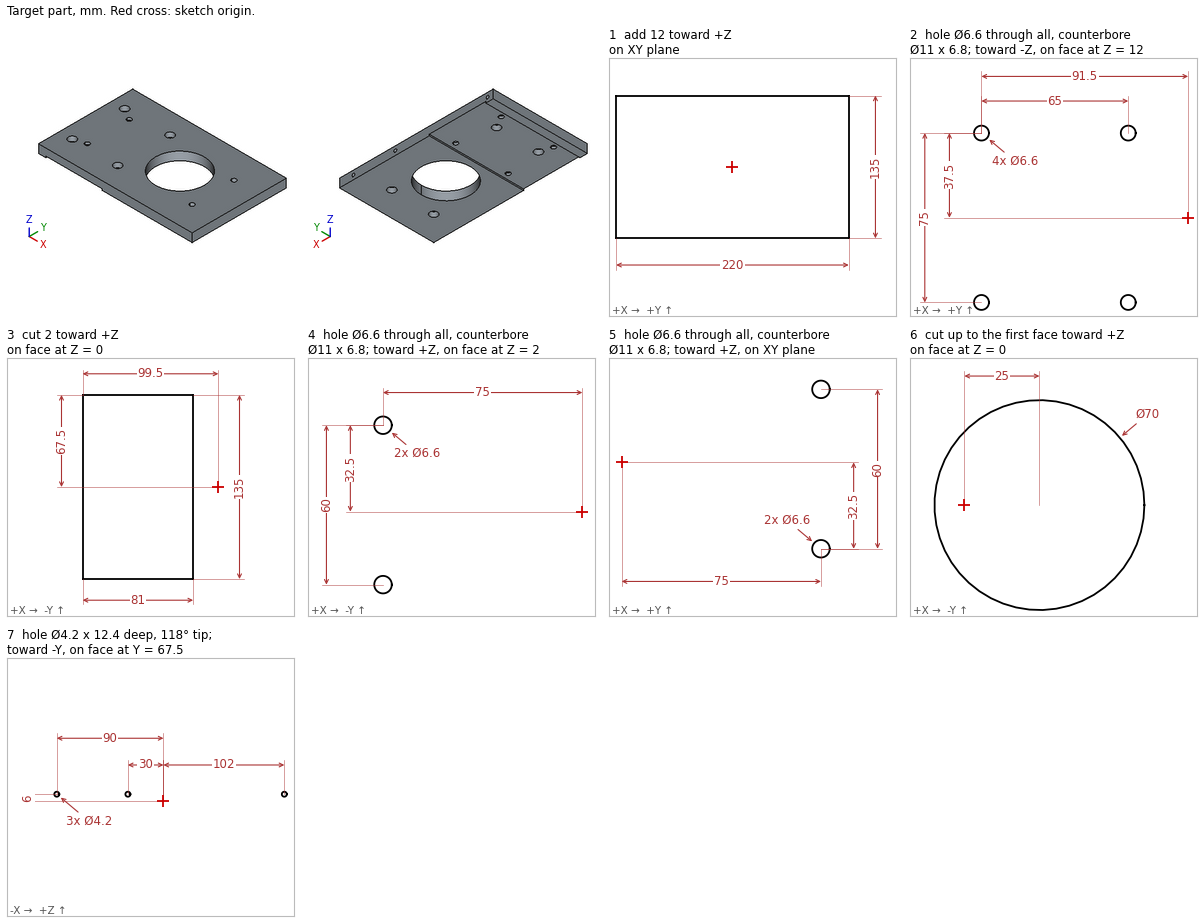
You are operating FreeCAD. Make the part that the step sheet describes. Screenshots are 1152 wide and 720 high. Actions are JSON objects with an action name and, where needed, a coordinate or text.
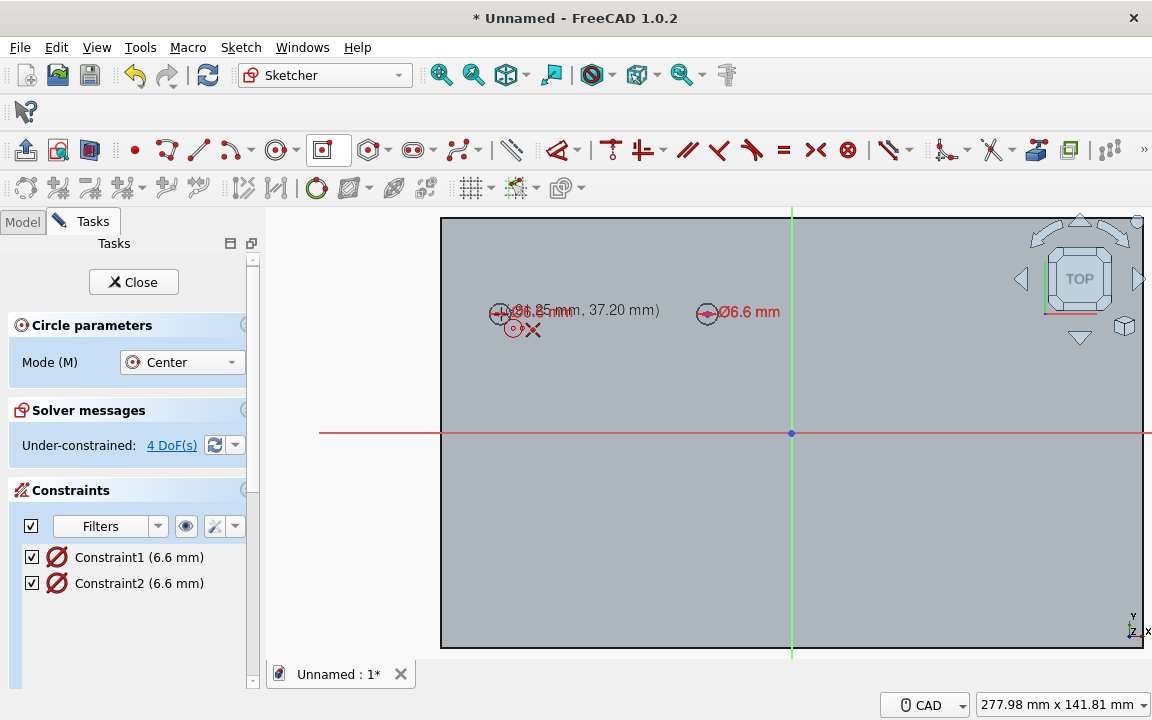
{"action": "scroll", "coordinate": [500, 553], "scroll_direction": "up", "scroll_amount": 4}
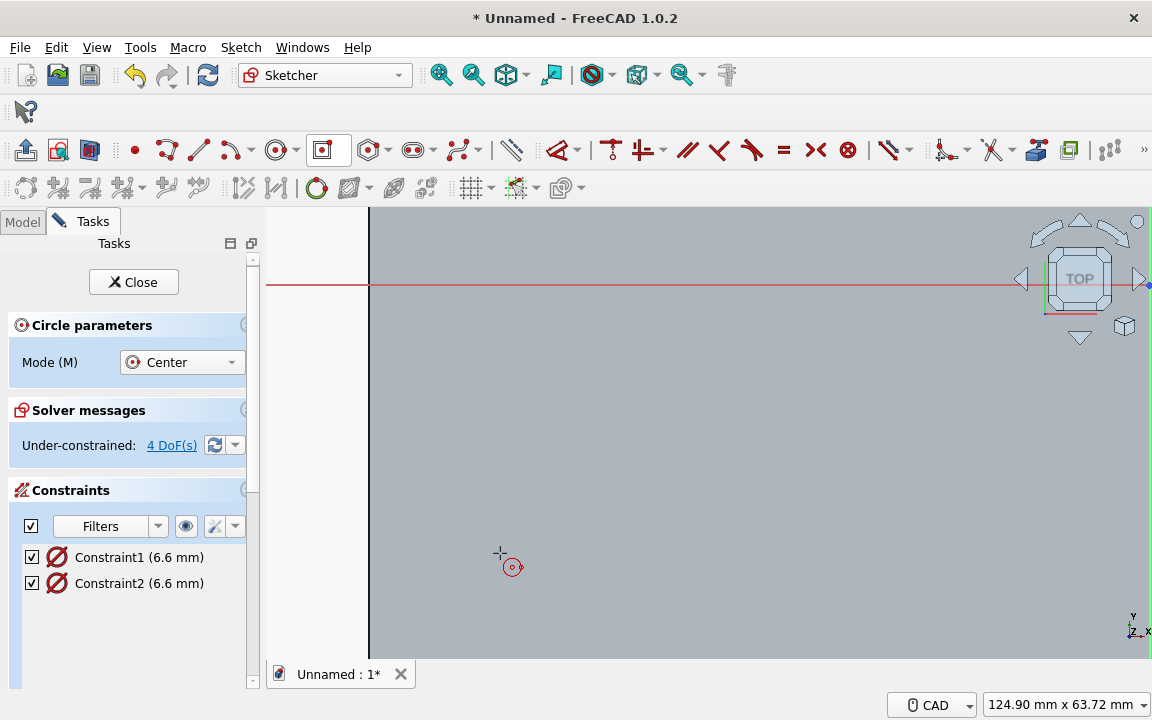
{"action": "left_click", "coordinate": [500, 551]}
{"action": "mouse_move", "coordinate": [517, 535]}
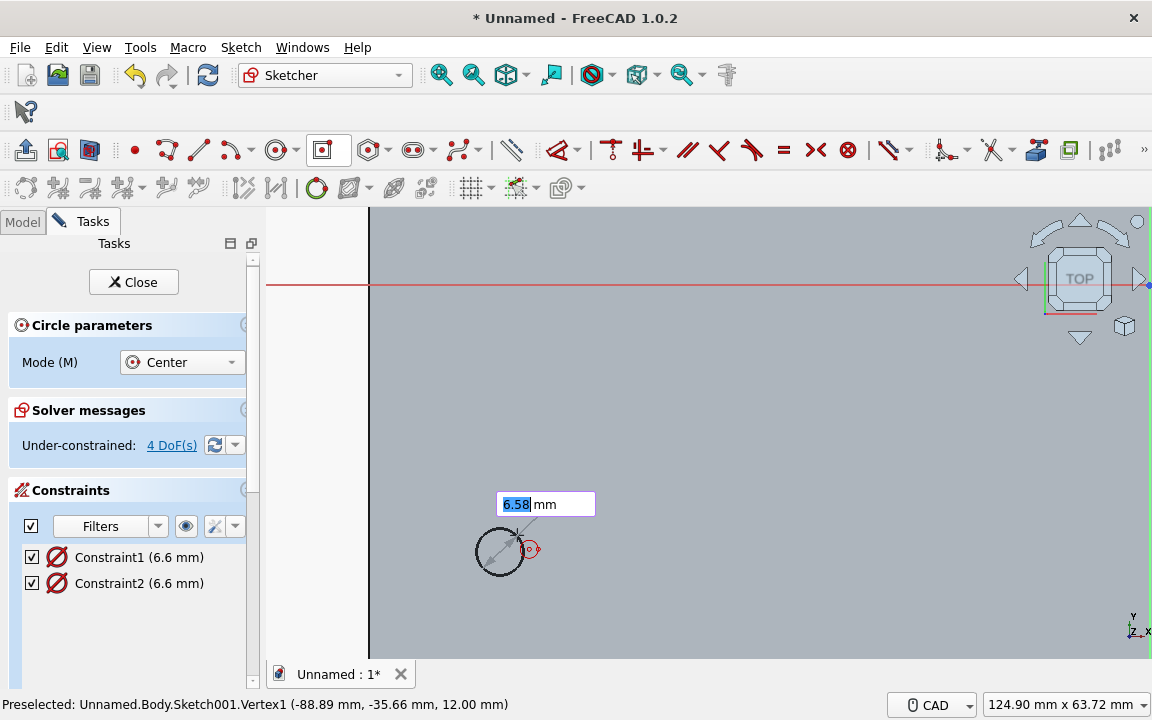
{"action": "type", "text": "6.6"}
{"action": "key", "text": "Return"}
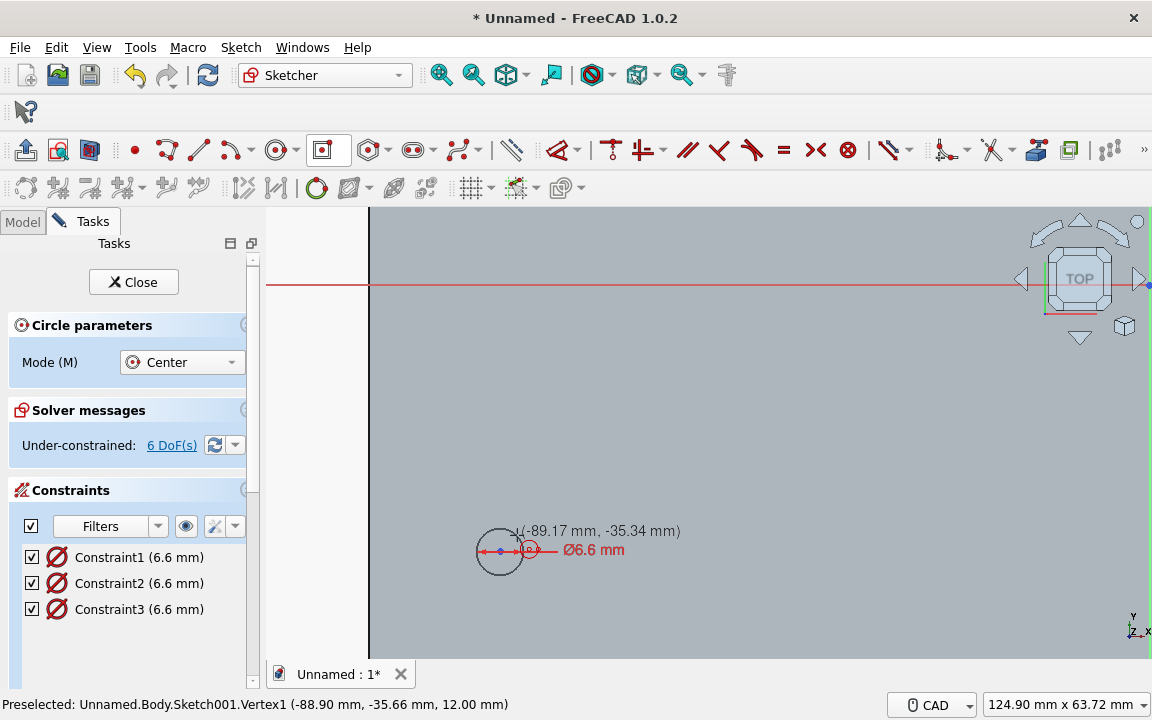
{"action": "left_click", "coordinate": [962, 551]}
{"action": "mouse_move", "coordinate": [978, 535]}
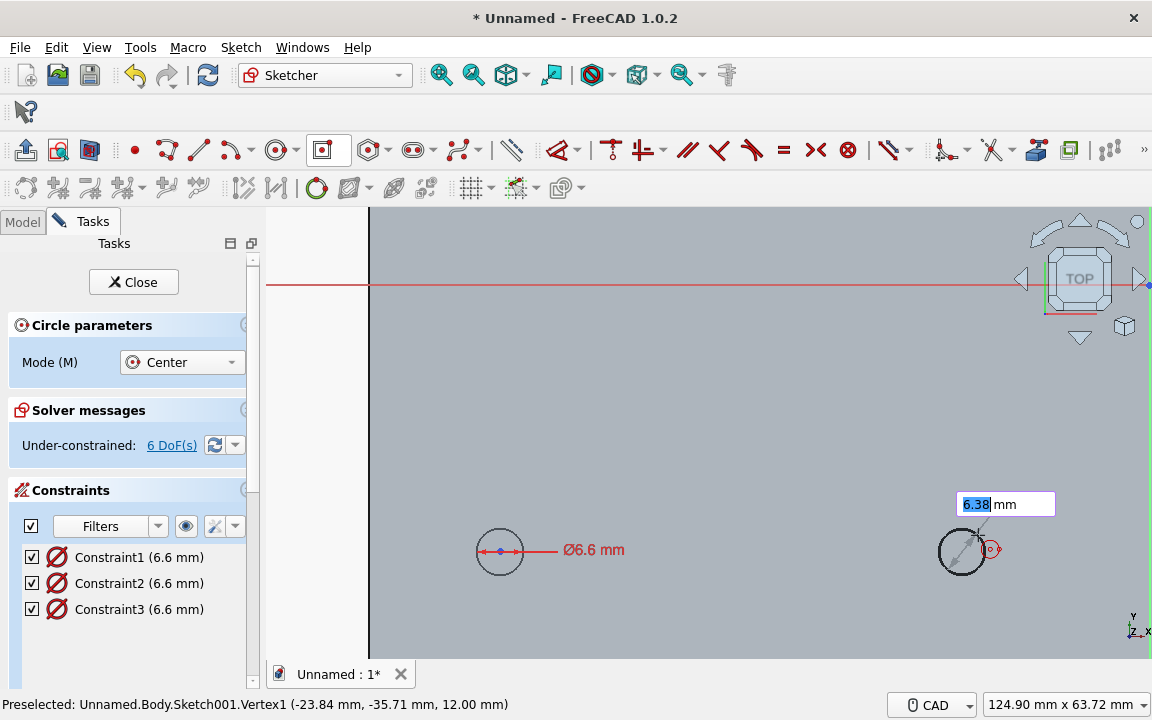
{"action": "type", "text": "6.6"}
{"action": "key", "text": "Return"}
{"action": "key", "text": "Escape"}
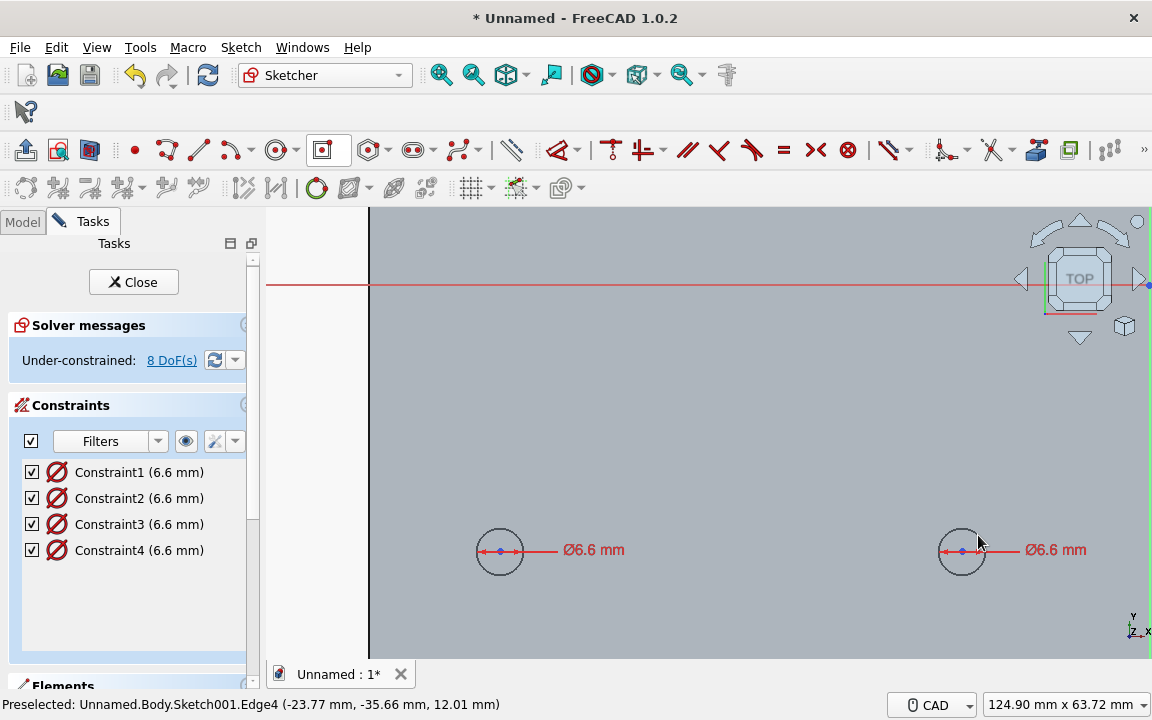
{"action": "scroll", "coordinate": [500, 554], "scroll_direction": "down", "scroll_amount": 4}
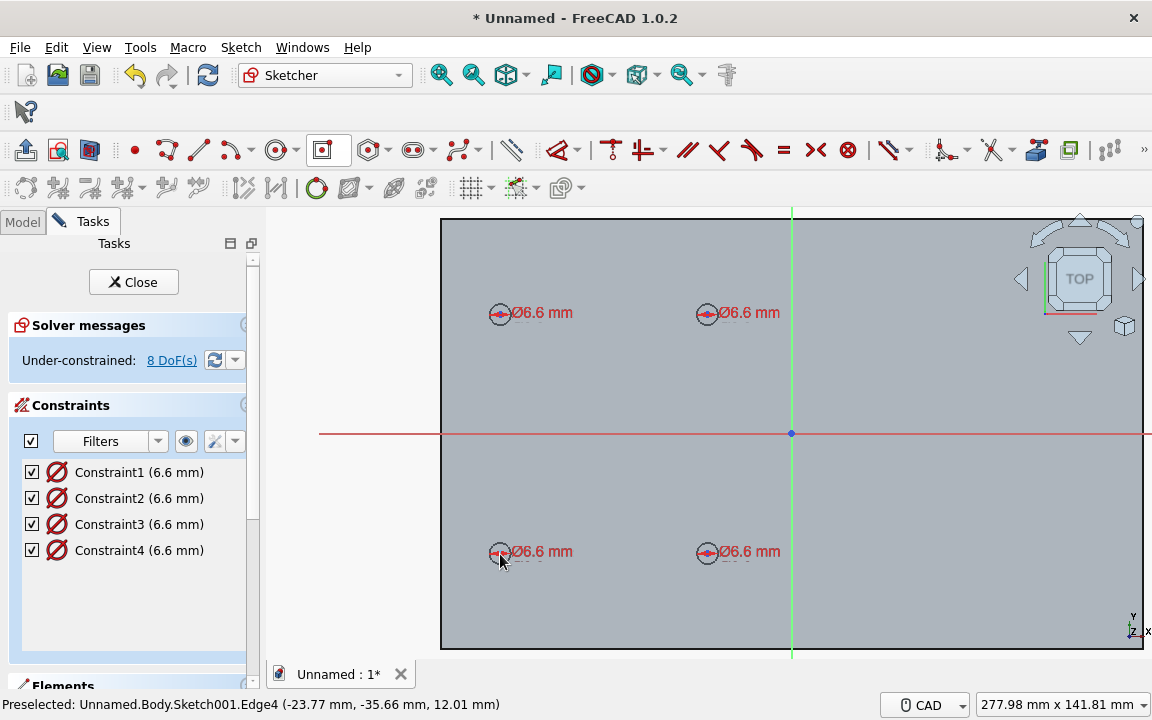
{"action": "left_click", "coordinate": [500, 315]}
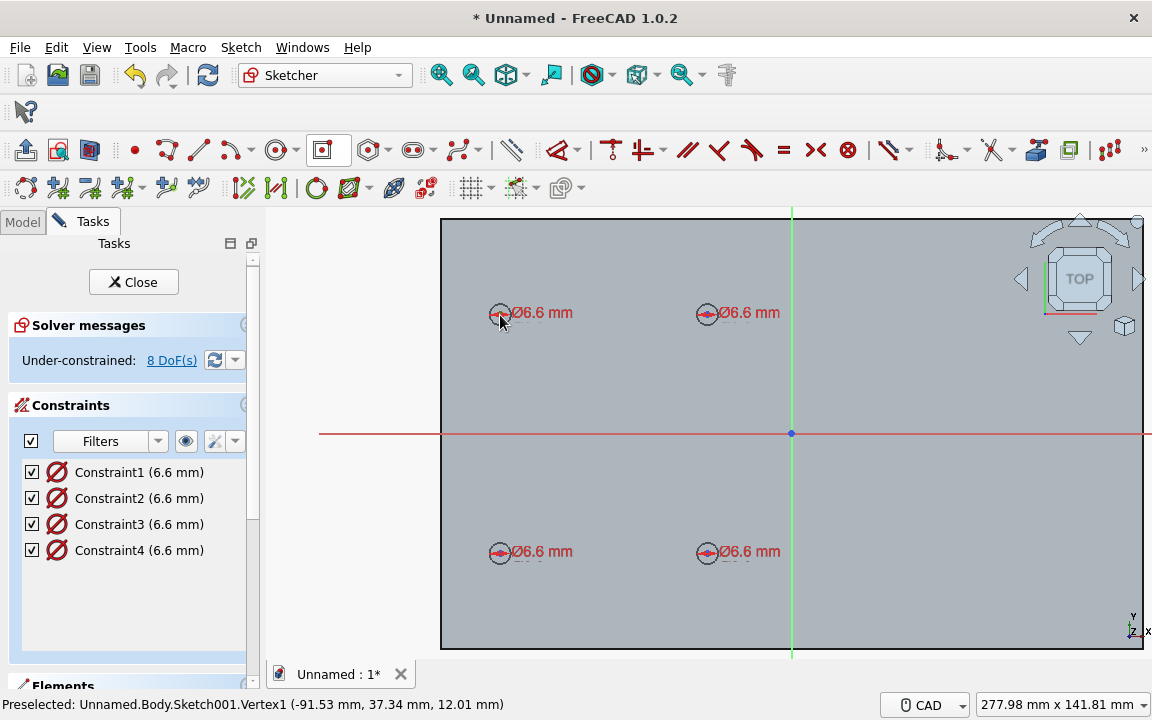
{"action": "left_click", "coordinate": [707, 315]}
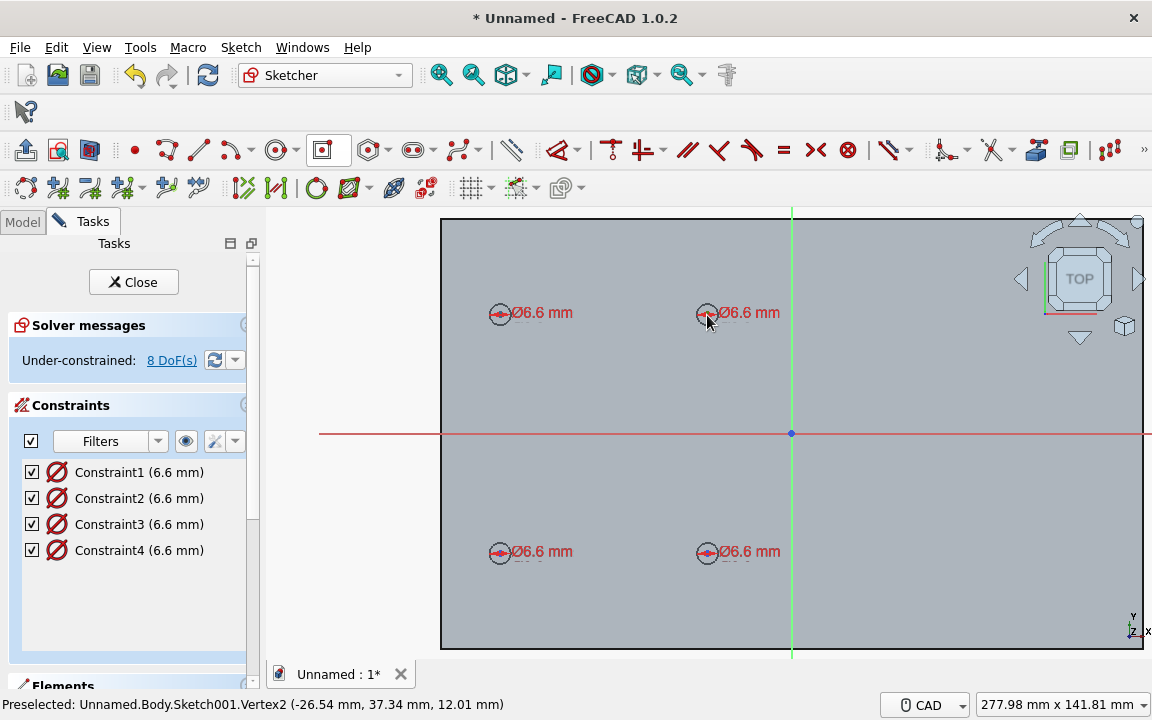
{"action": "key", "text": "h"}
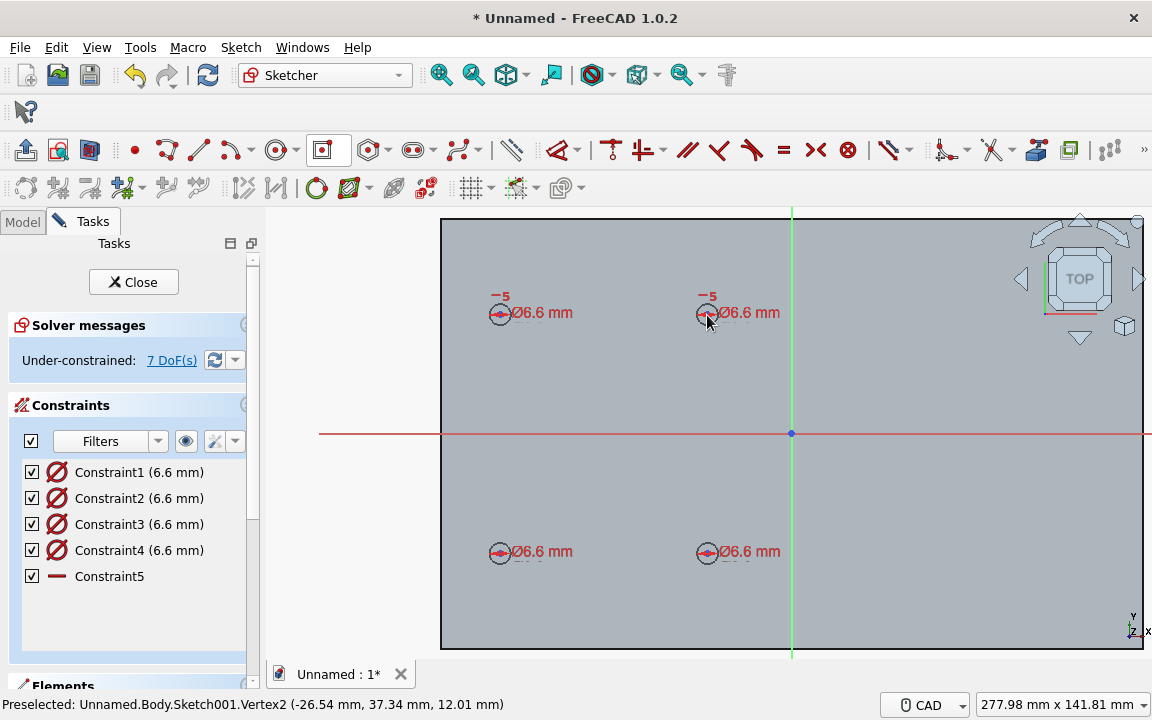
{"action": "left_click", "coordinate": [500, 315]}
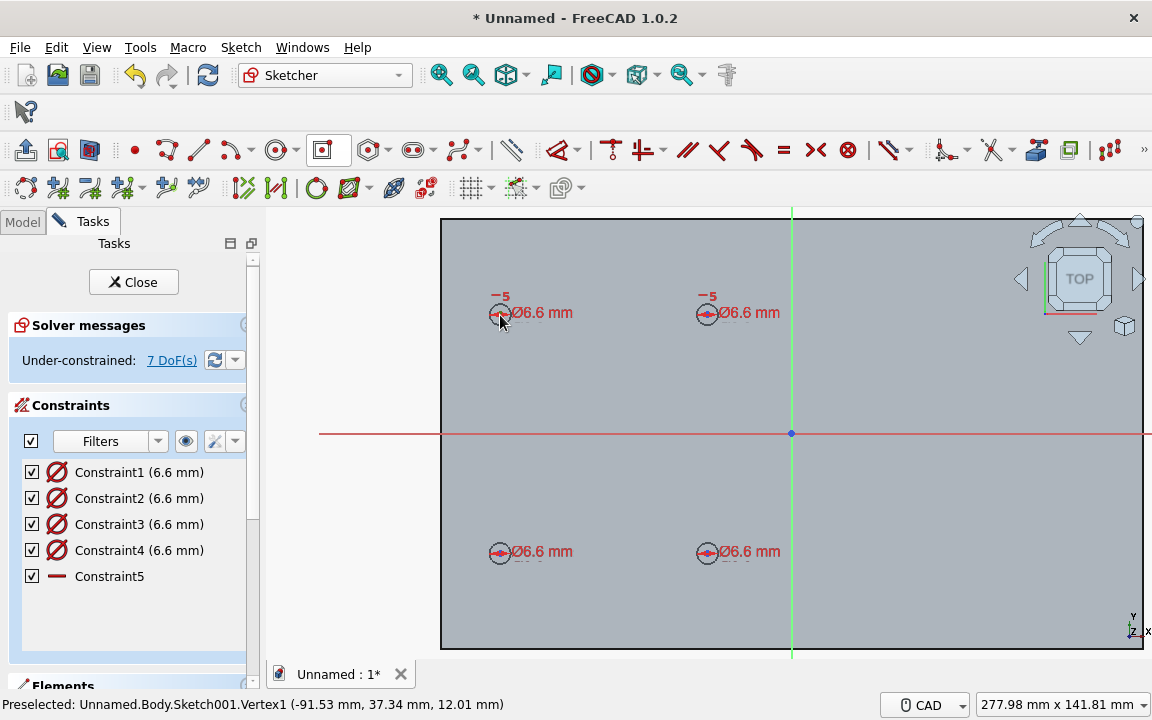
{"action": "left_click", "coordinate": [500, 554]}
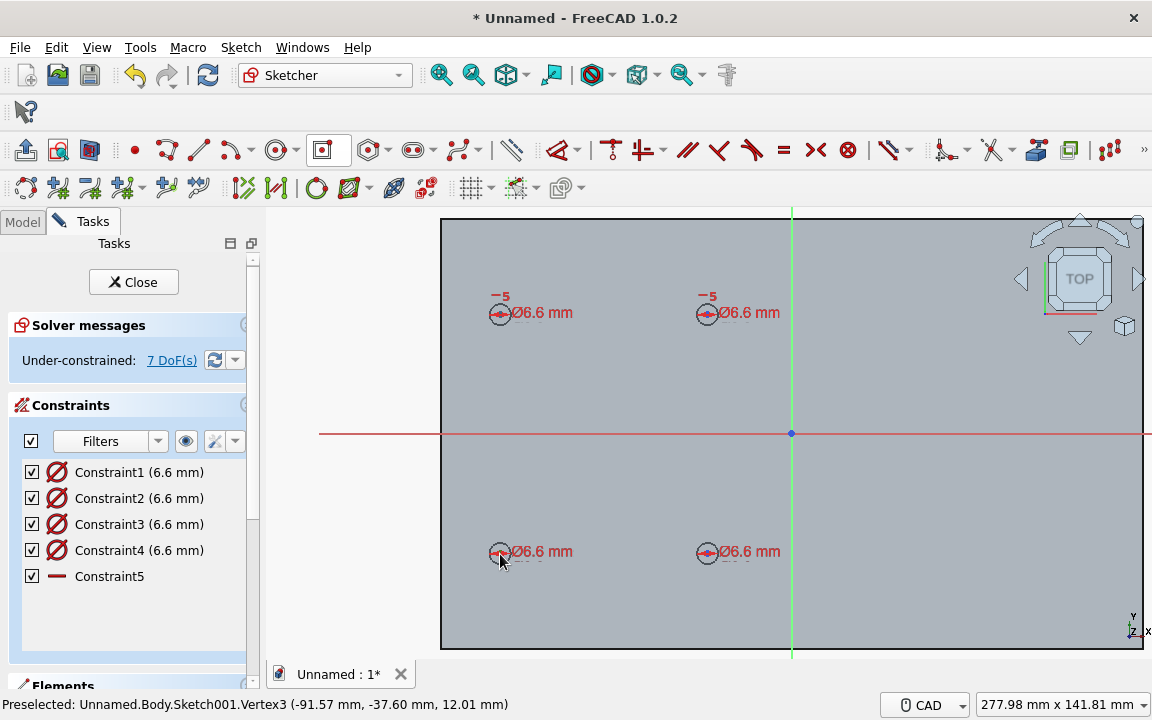
{"action": "left_click", "coordinate": [666, 150]}